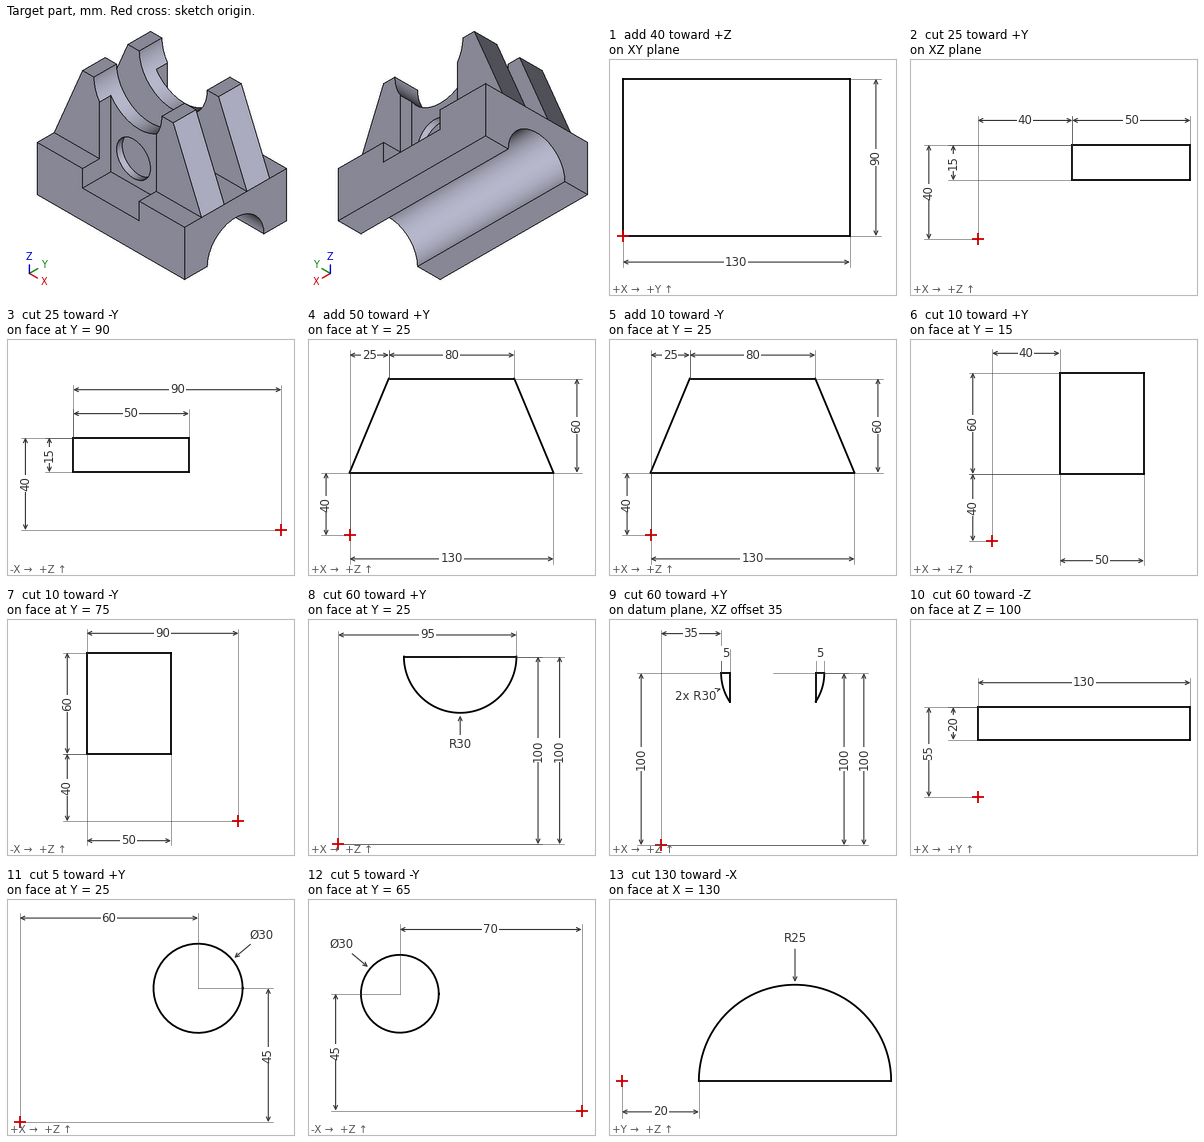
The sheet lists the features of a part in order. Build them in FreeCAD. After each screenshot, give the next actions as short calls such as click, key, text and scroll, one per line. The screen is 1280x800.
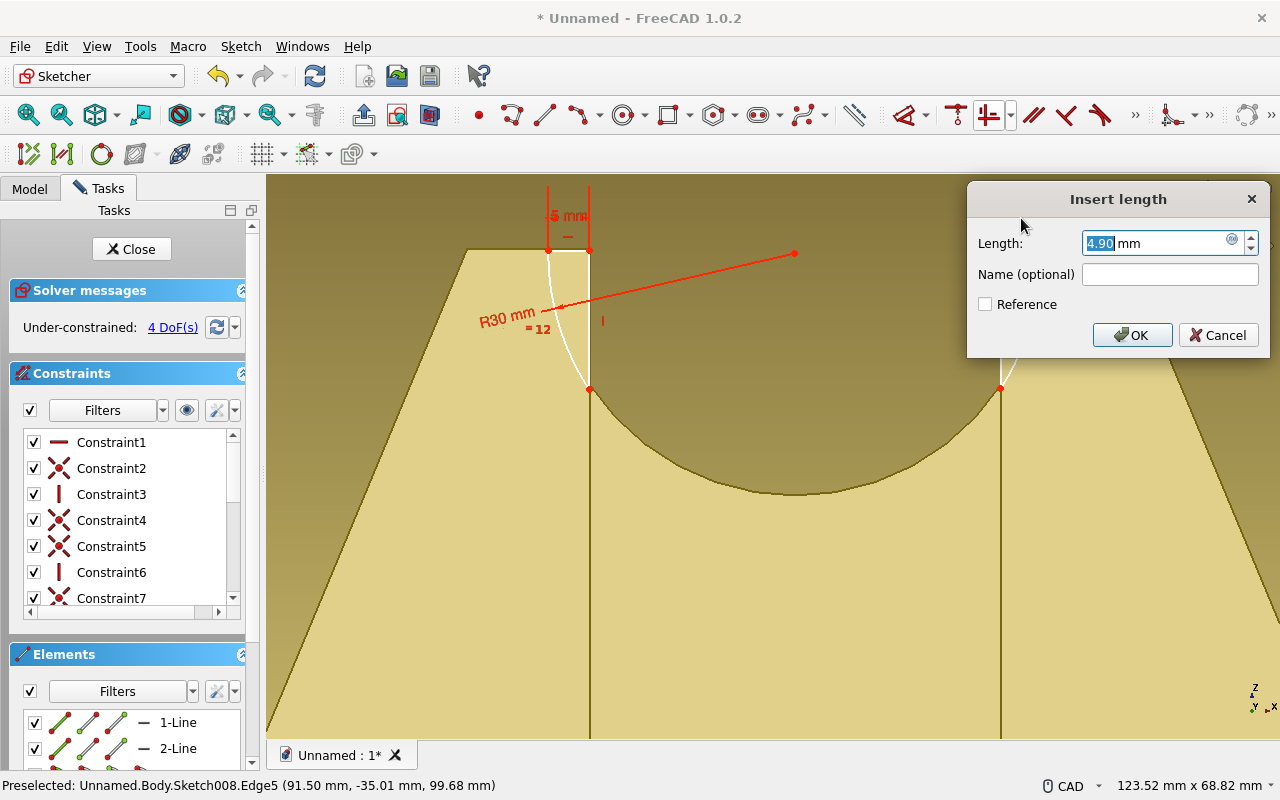
text(5)
key(Return)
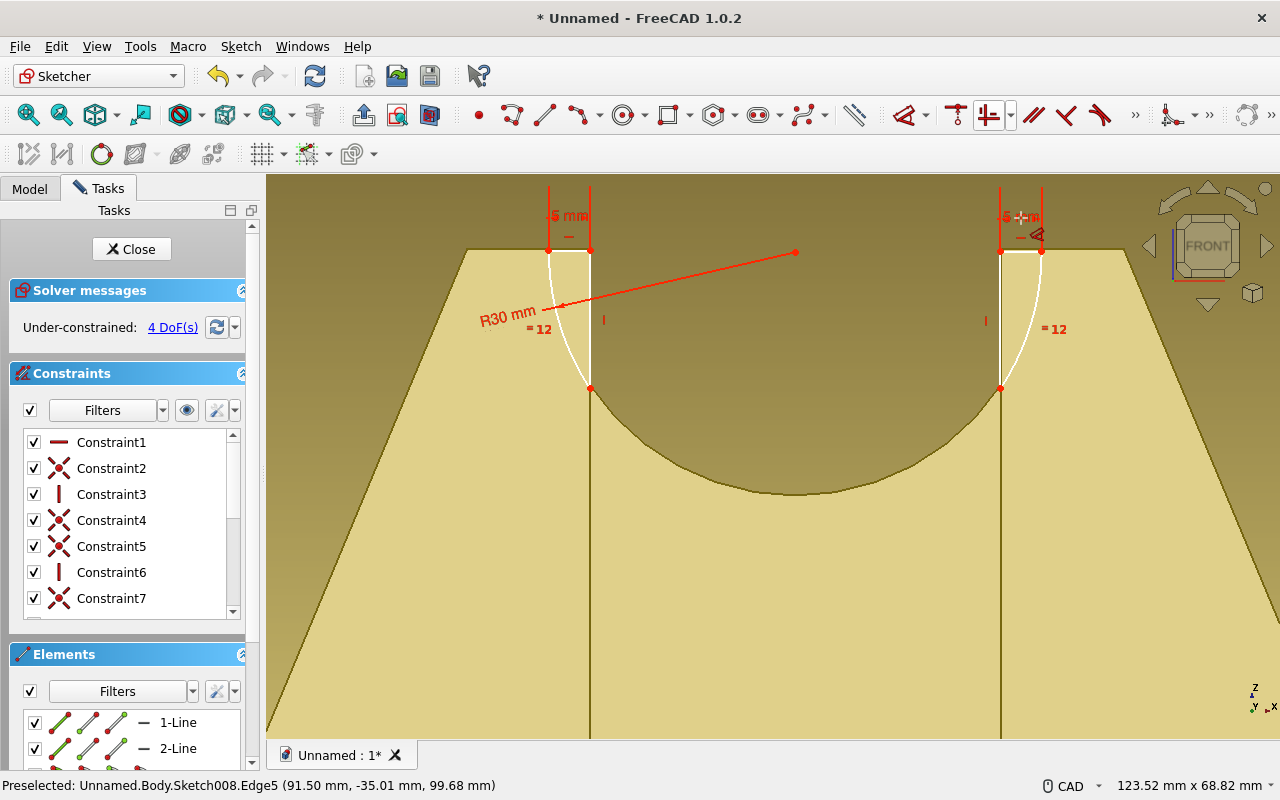
click(549, 251)
click(421, 217)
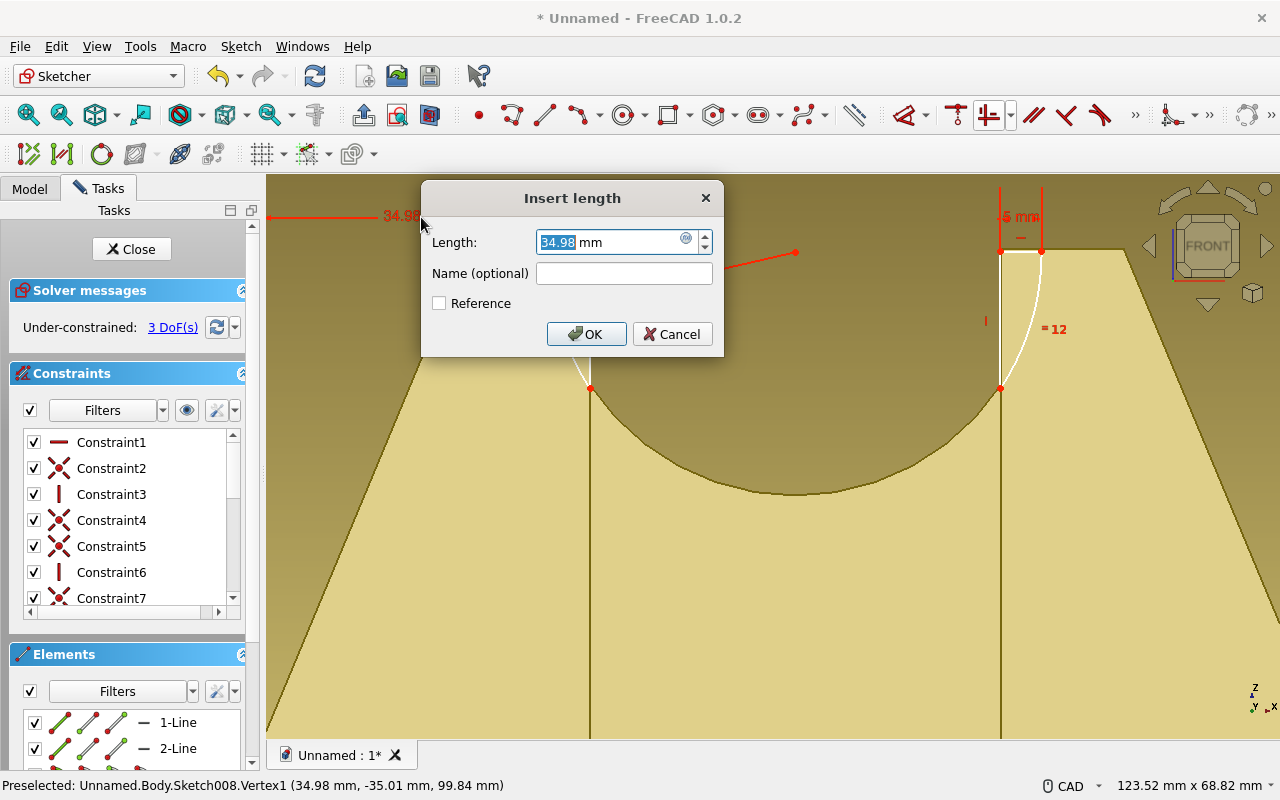
text(35)
key(Return)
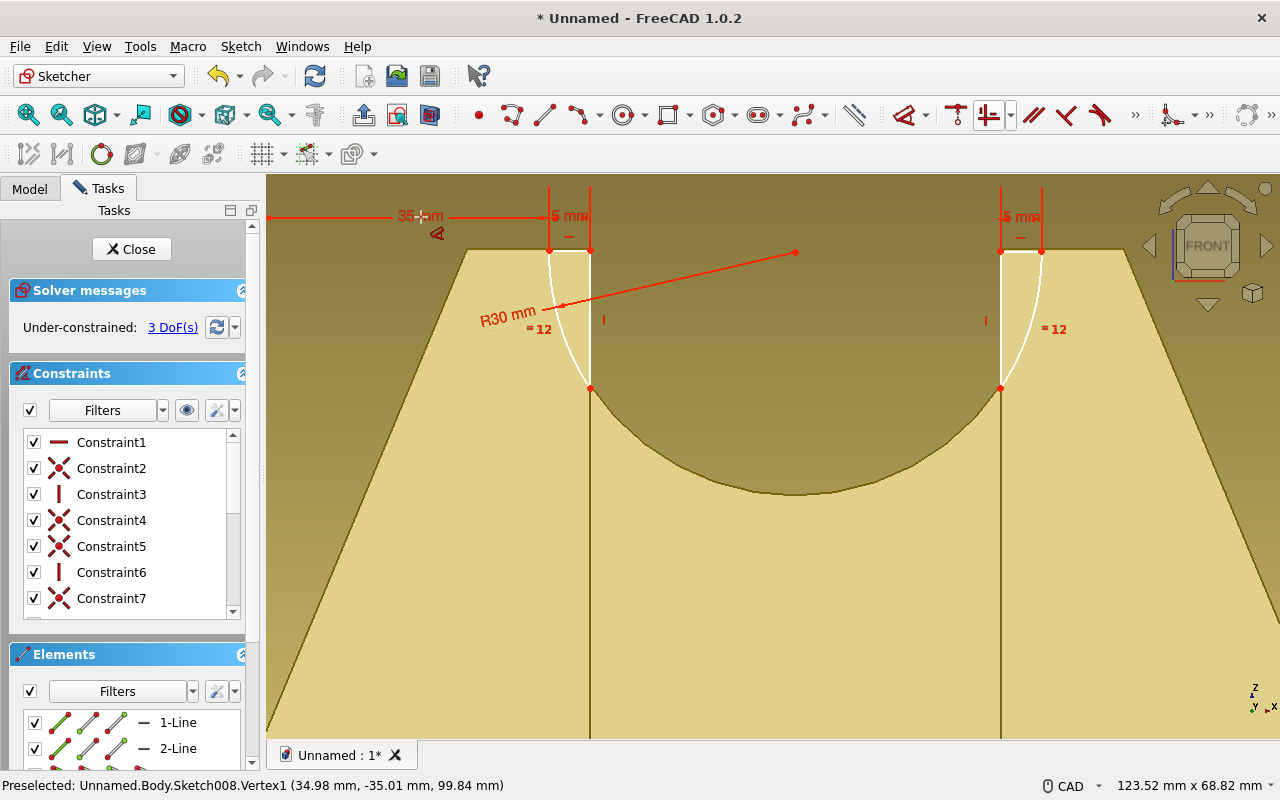
click(549, 251)
click(583, 481)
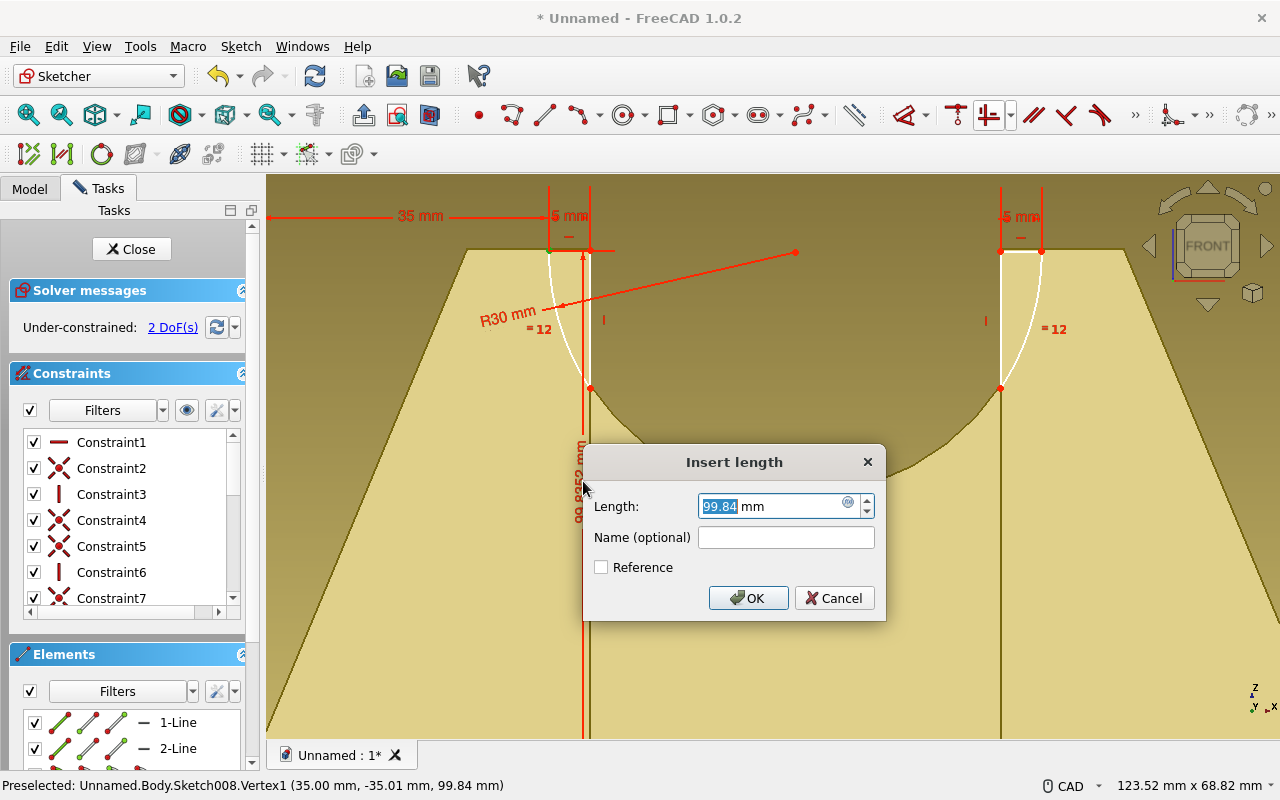
text(100)
key(Return)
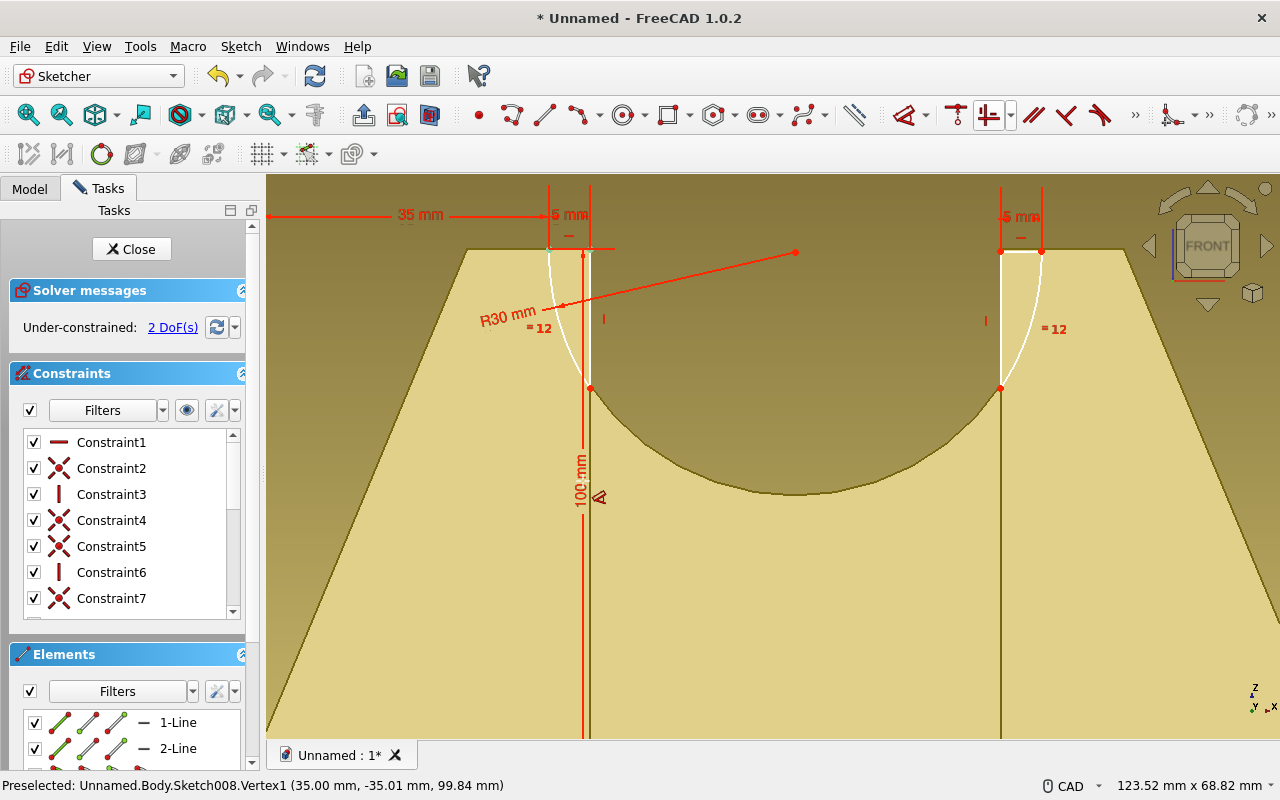
click(1001, 252)
click(1035, 481)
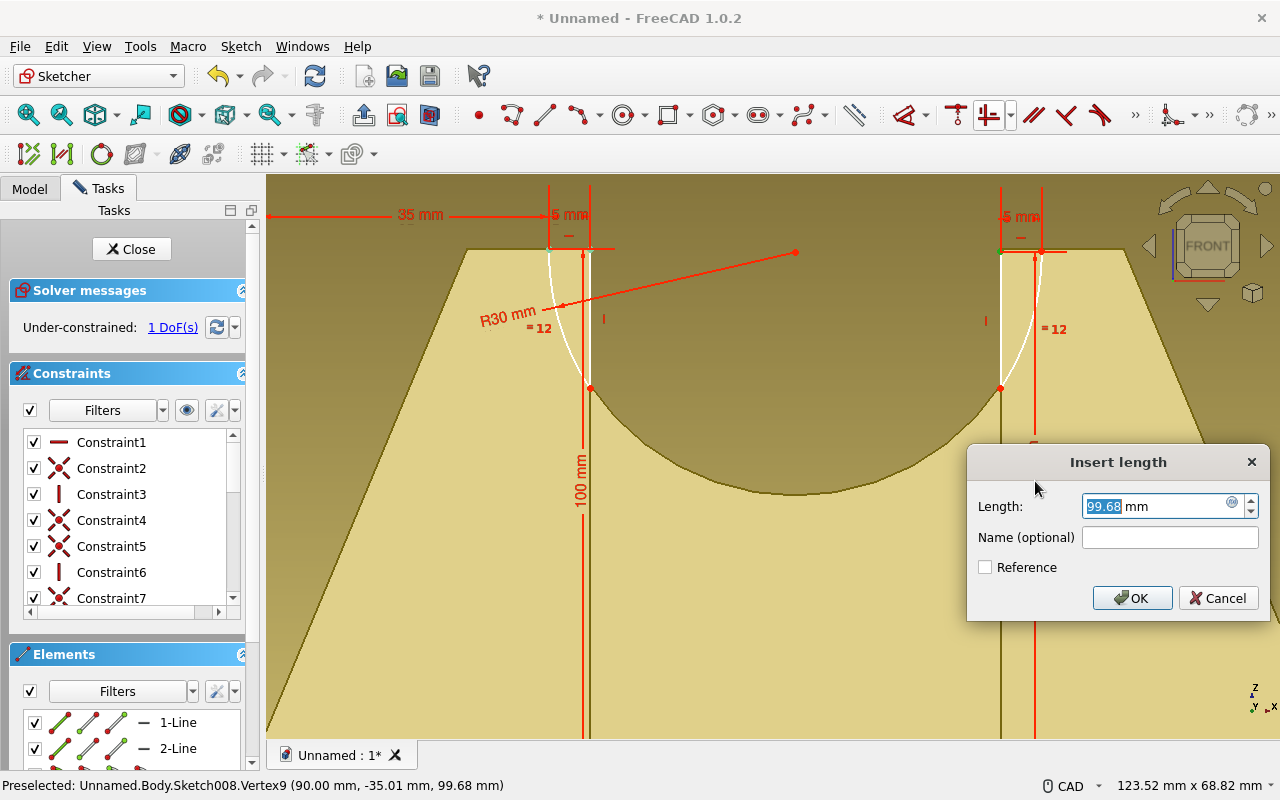
text(100)
key(Return)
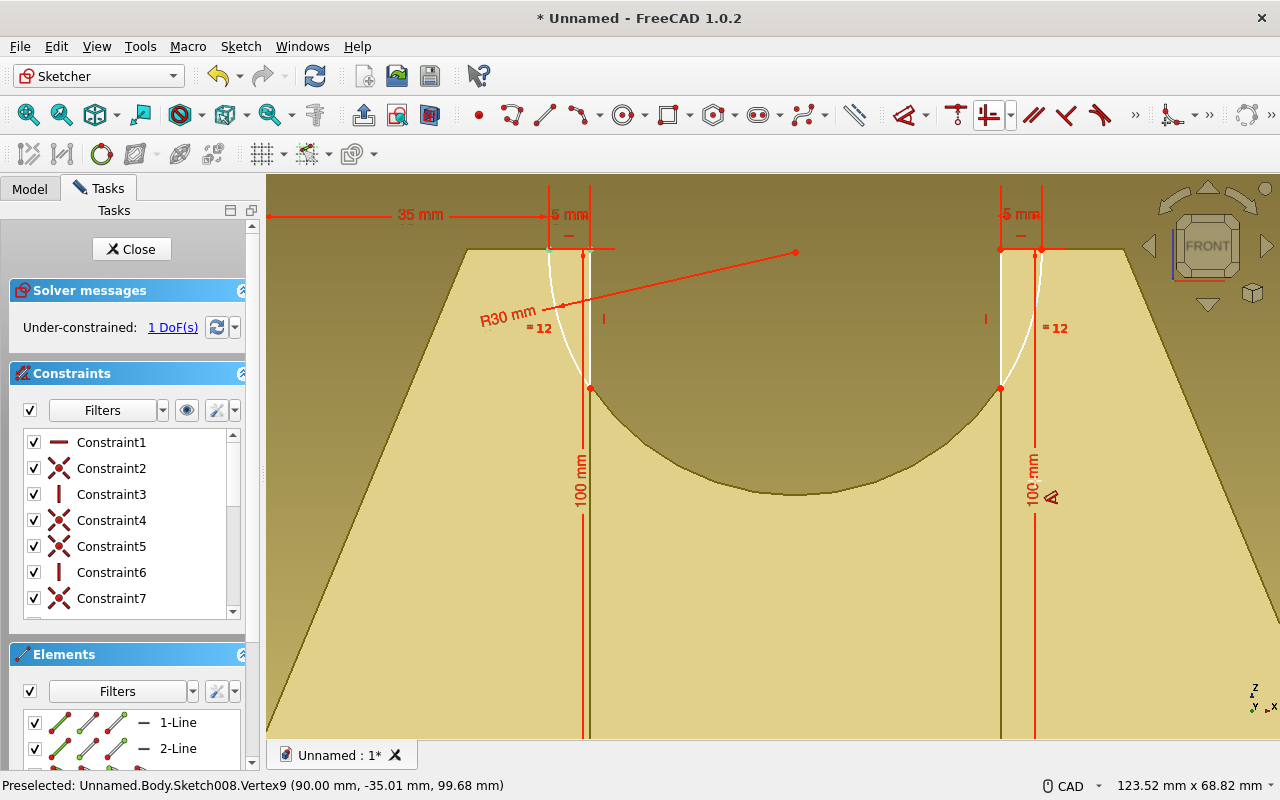
click(795, 252)
click(829, 482)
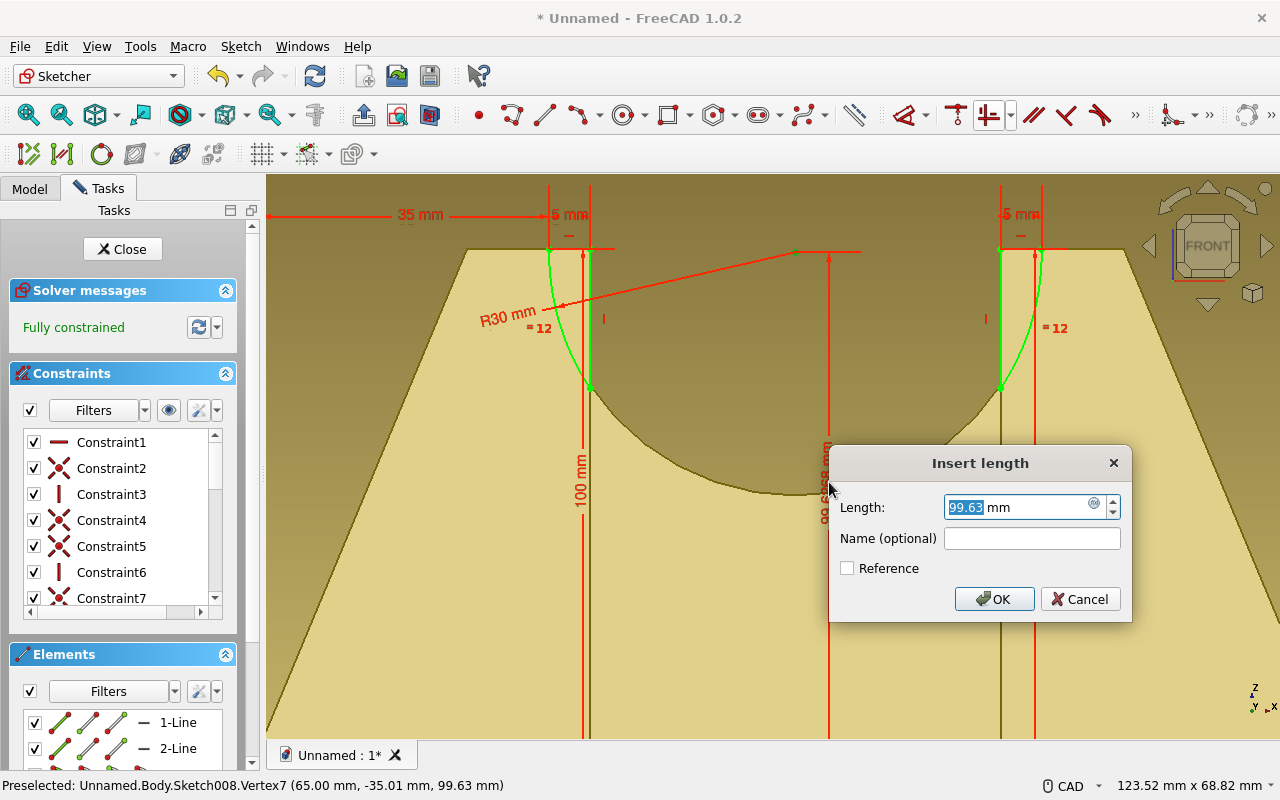
text(100)
key(Return)
key(Escape)